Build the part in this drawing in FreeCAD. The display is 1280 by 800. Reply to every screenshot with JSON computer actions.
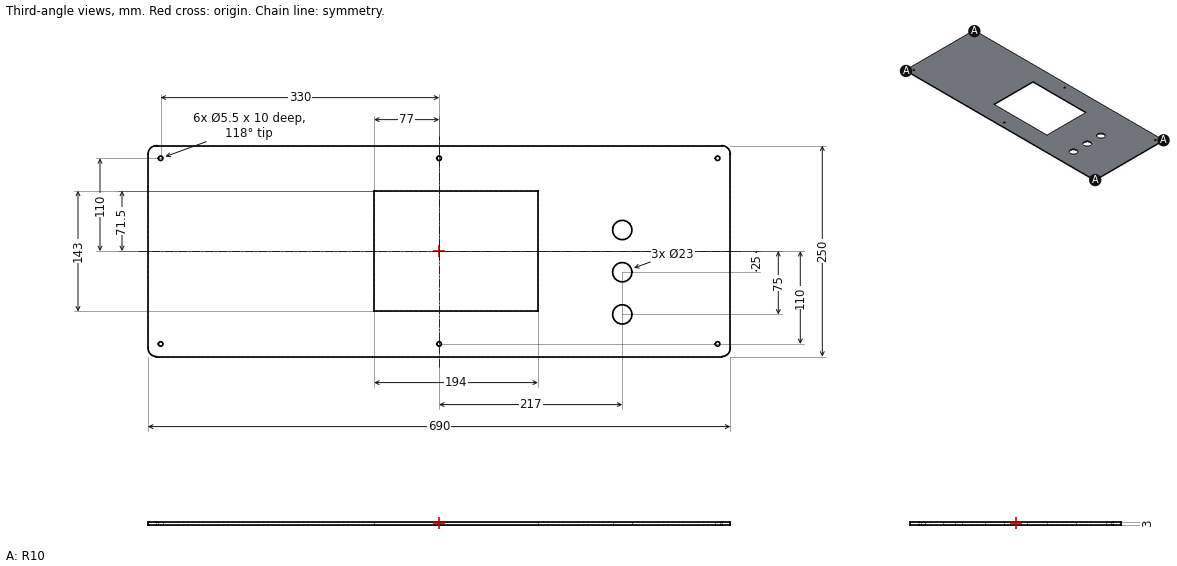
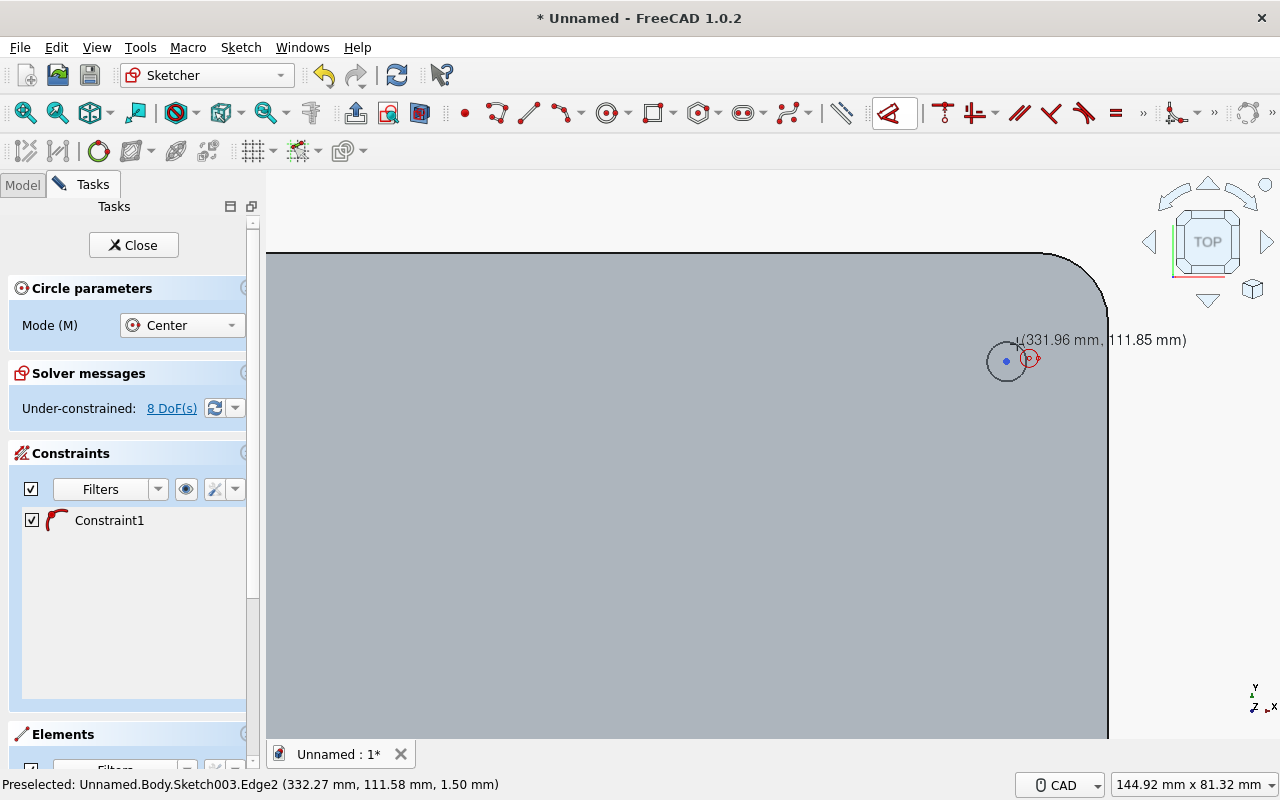
{"action": "scroll", "coordinate": [1019, 349], "scroll_direction": "down", "scroll_amount": 10}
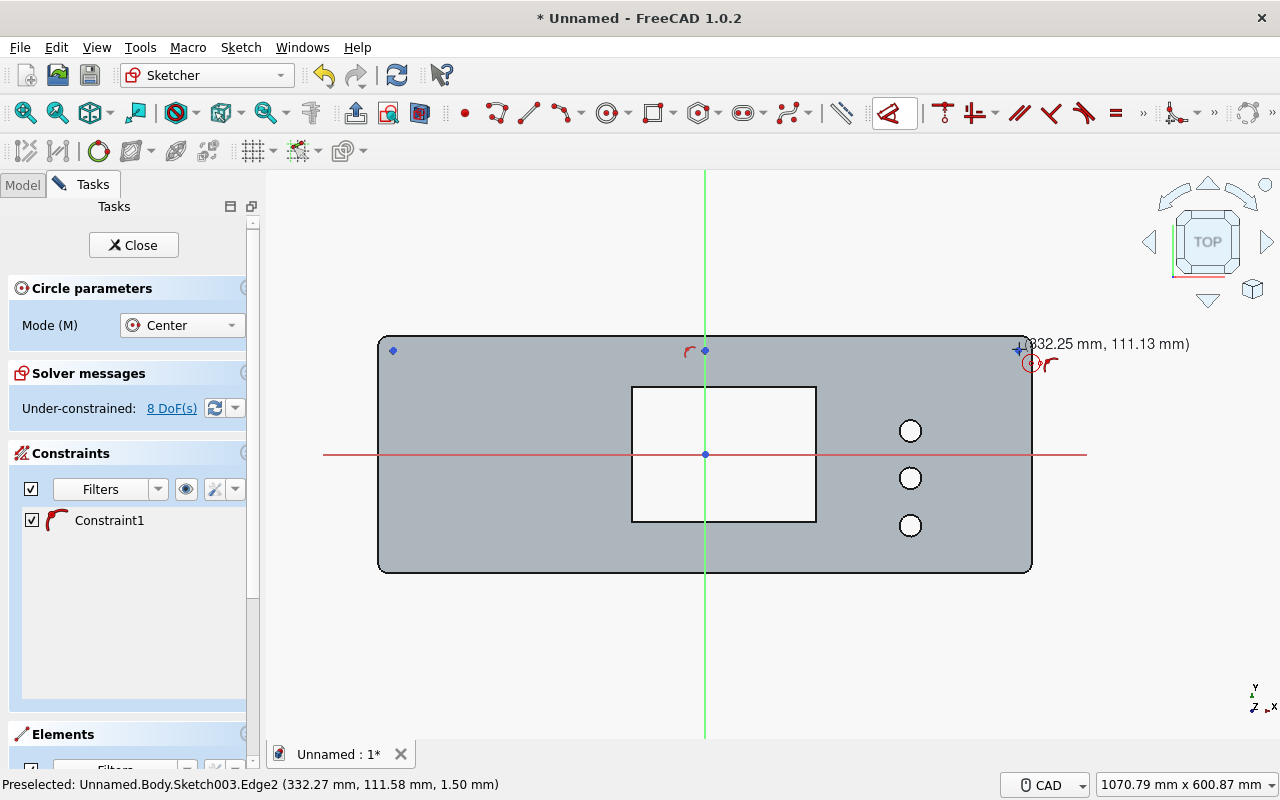
{"action": "scroll", "coordinate": [1018, 559], "scroll_direction": "up", "scroll_amount": 11}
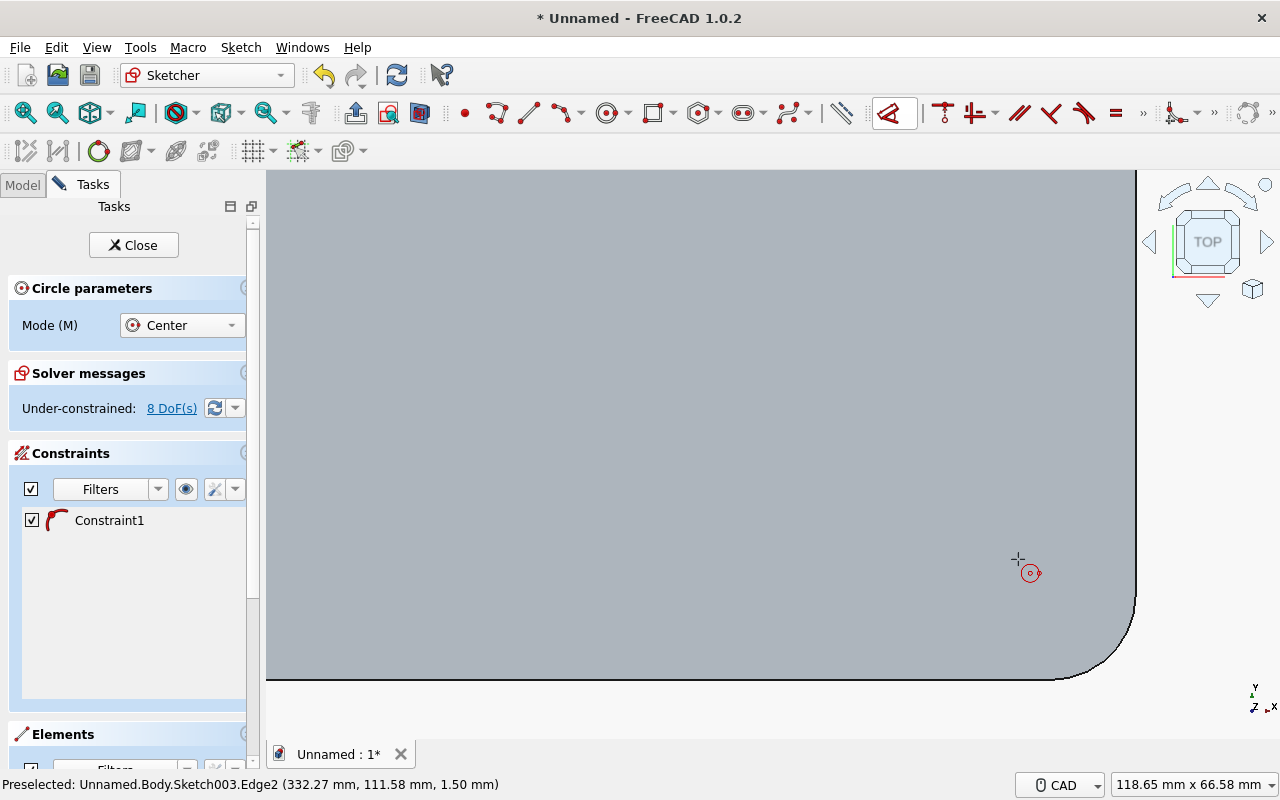
{"action": "scroll", "coordinate": [1018, 560], "scroll_direction": "down", "scroll_amount": 11}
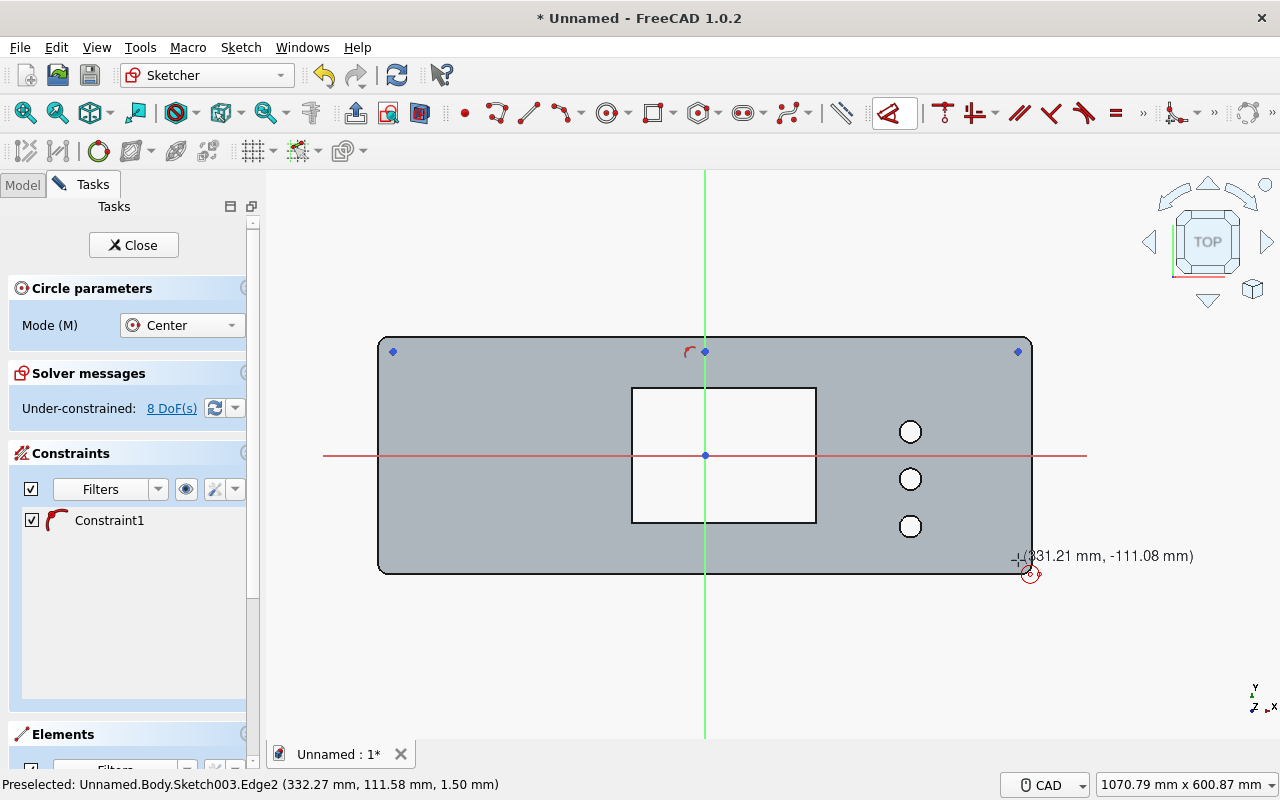
{"action": "left_click", "coordinate": [1018, 560]}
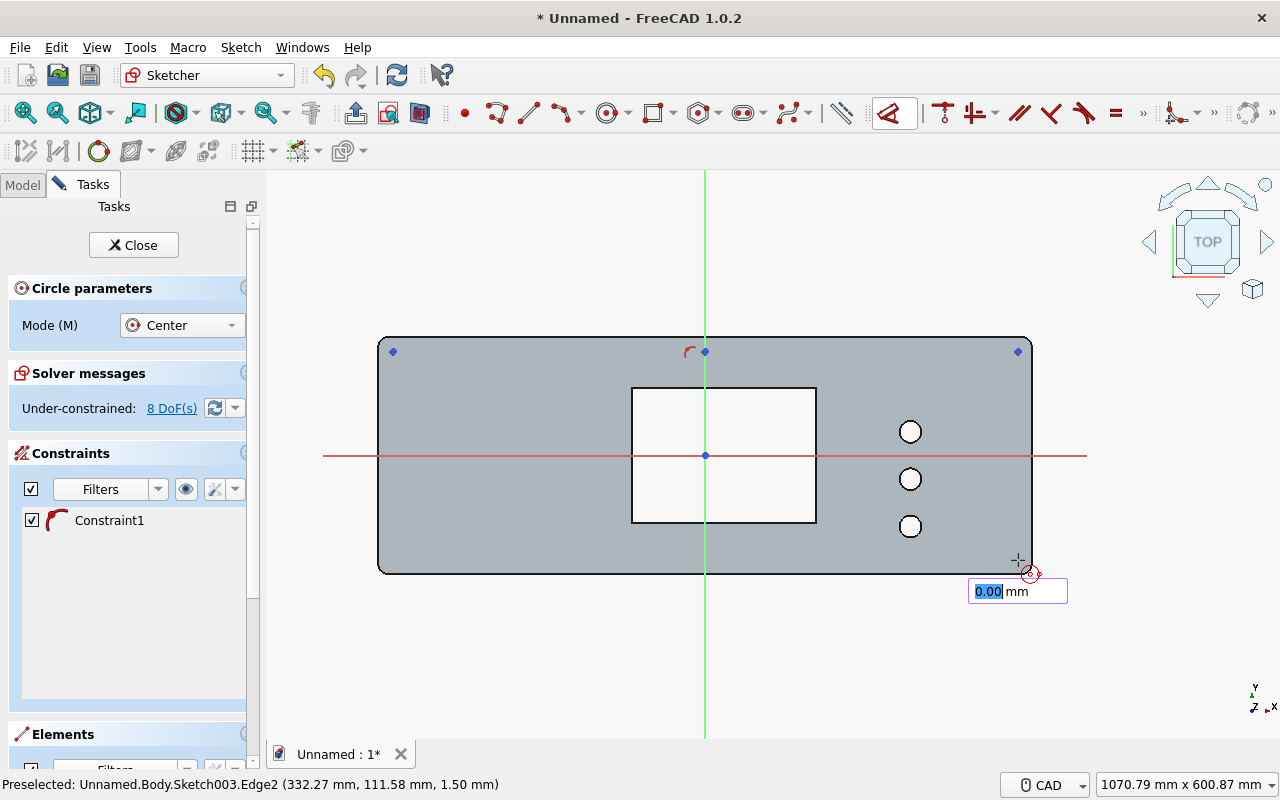
{"action": "scroll", "coordinate": [1019, 558], "scroll_direction": "up", "scroll_amount": 10}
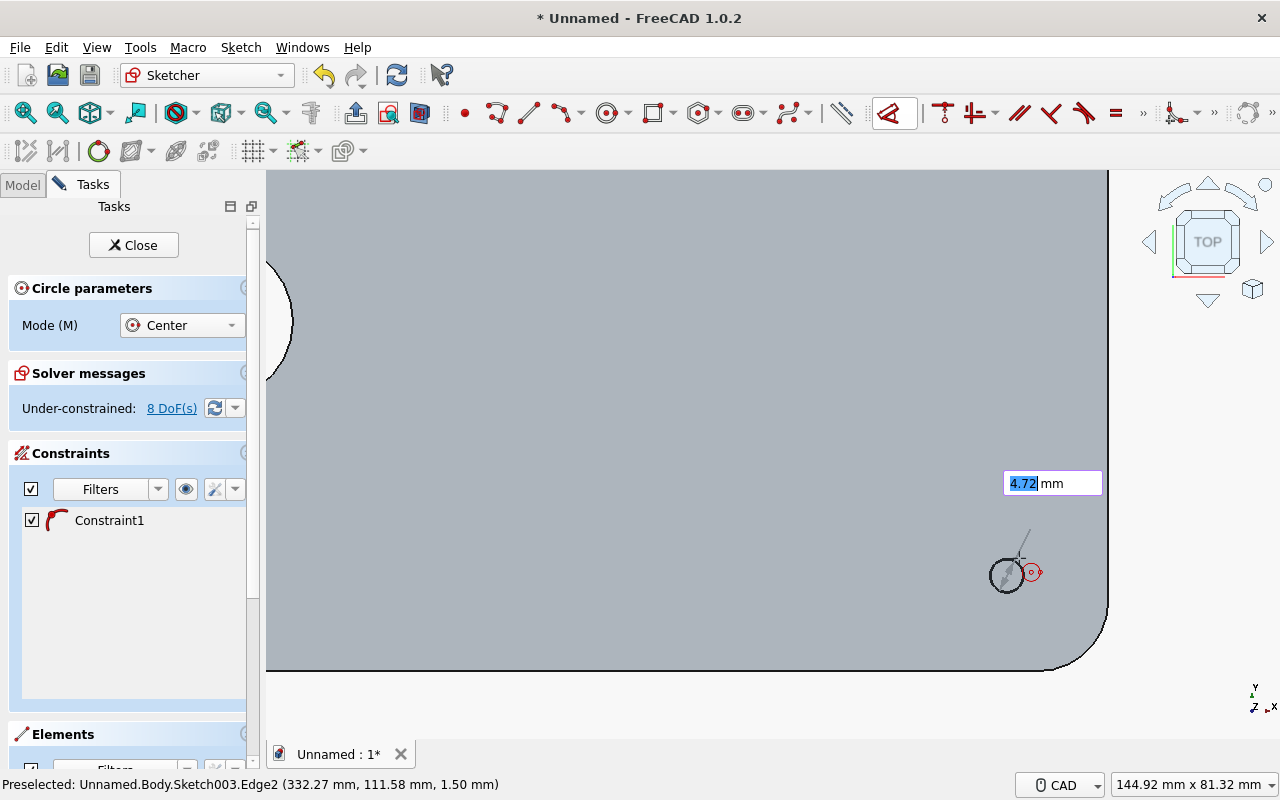
{"action": "left_click", "coordinate": [1017, 553]}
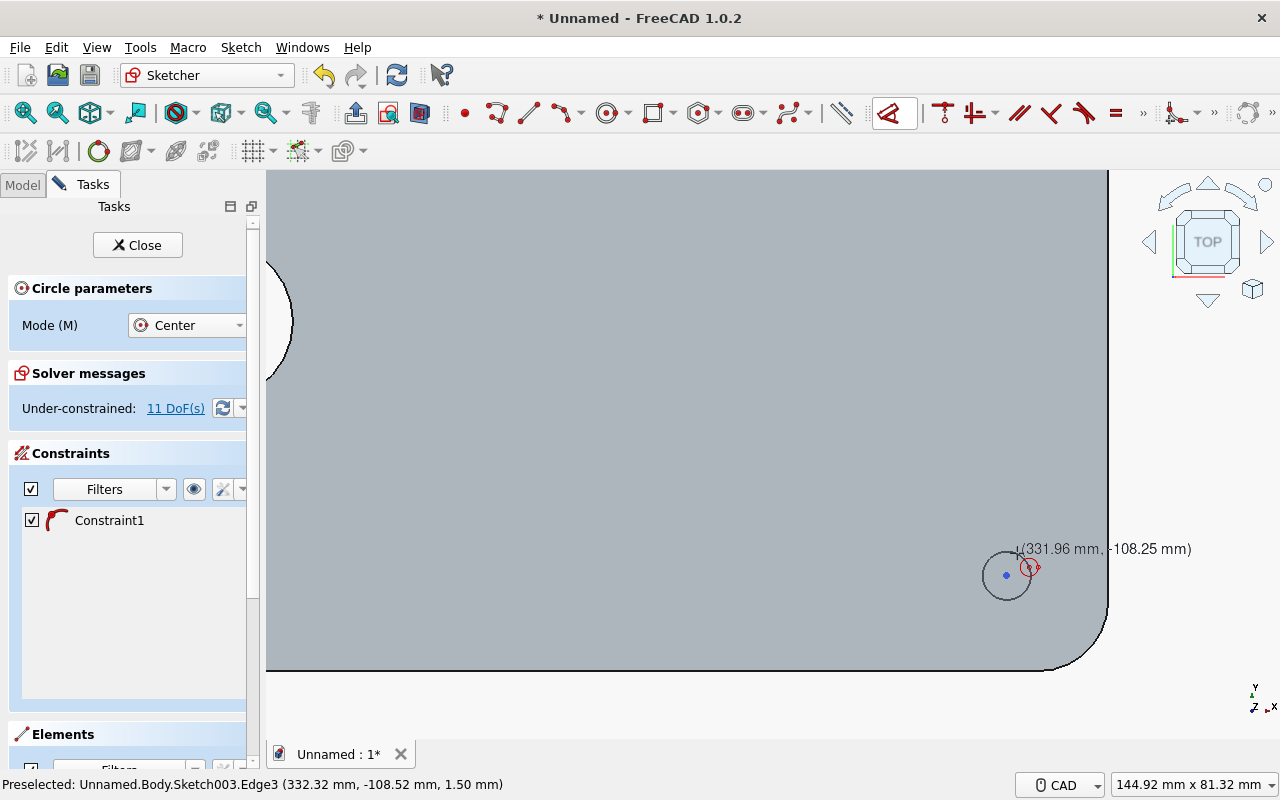
{"action": "scroll", "coordinate": [1019, 557], "scroll_direction": "down", "scroll_amount": 10}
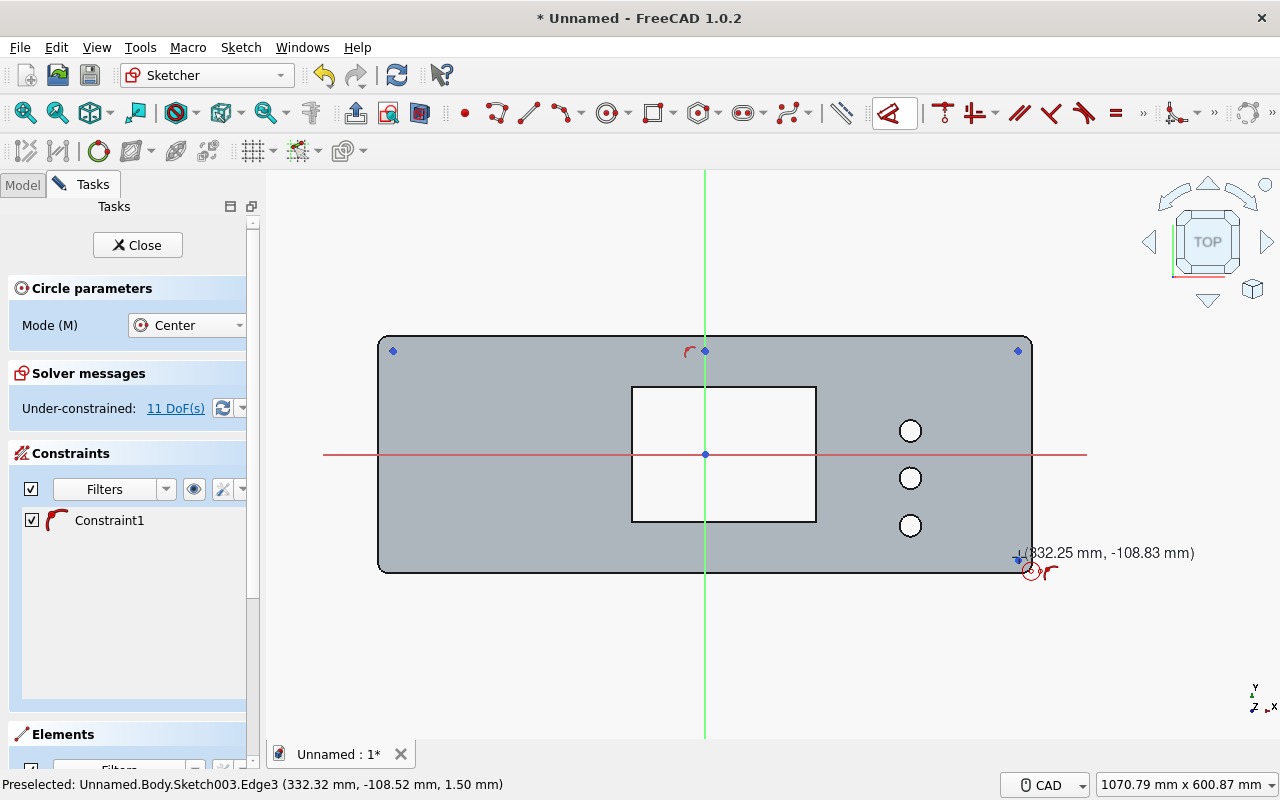
{"action": "scroll", "coordinate": [705, 559], "scroll_direction": "up", "scroll_amount": 11}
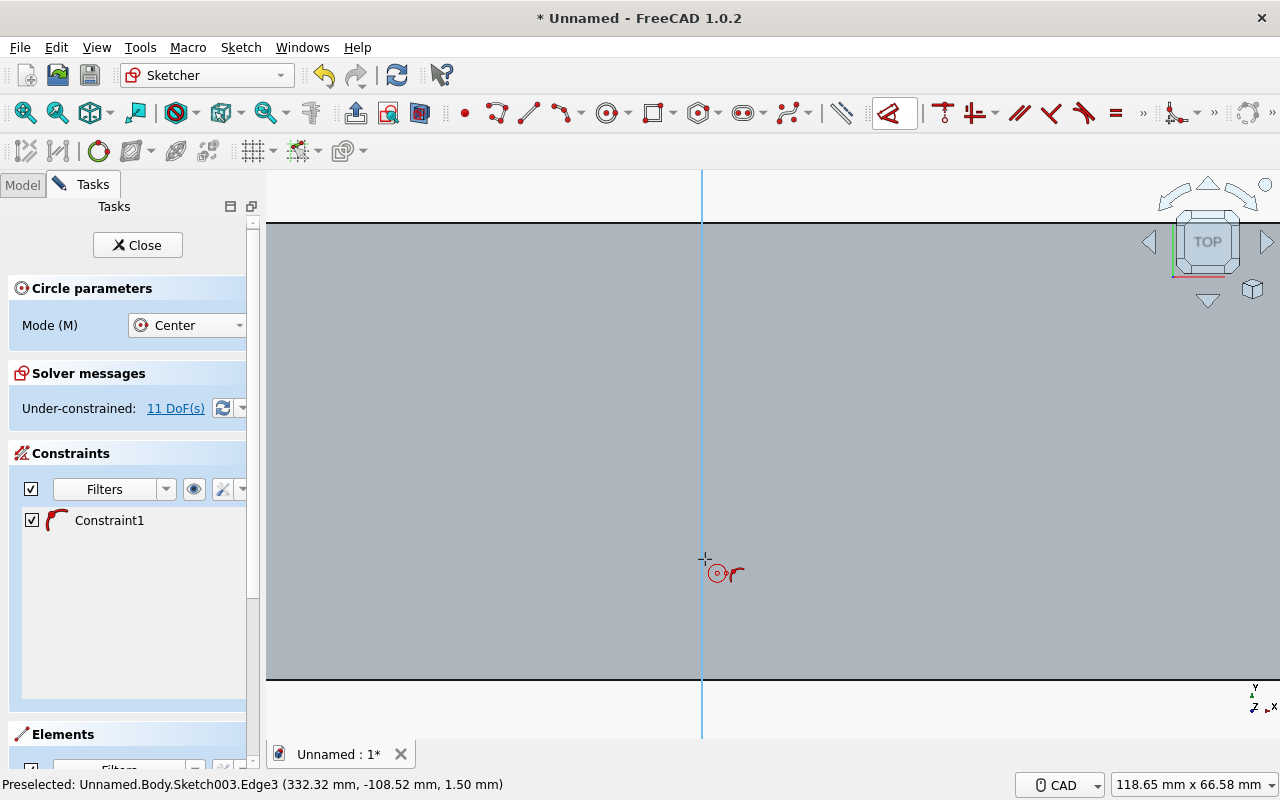
{"action": "scroll", "coordinate": [705, 559], "scroll_direction": "down", "scroll_amount": 11}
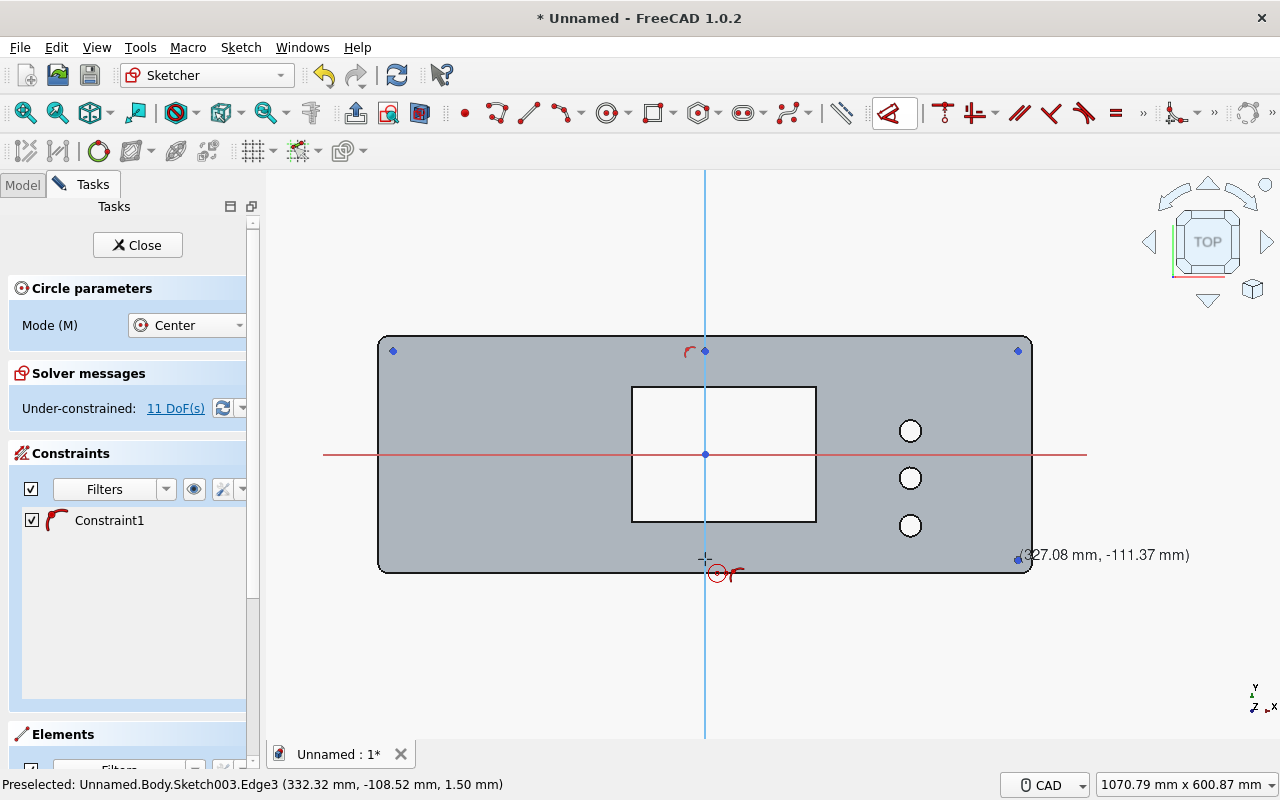
{"action": "left_click", "coordinate": [705, 559]}